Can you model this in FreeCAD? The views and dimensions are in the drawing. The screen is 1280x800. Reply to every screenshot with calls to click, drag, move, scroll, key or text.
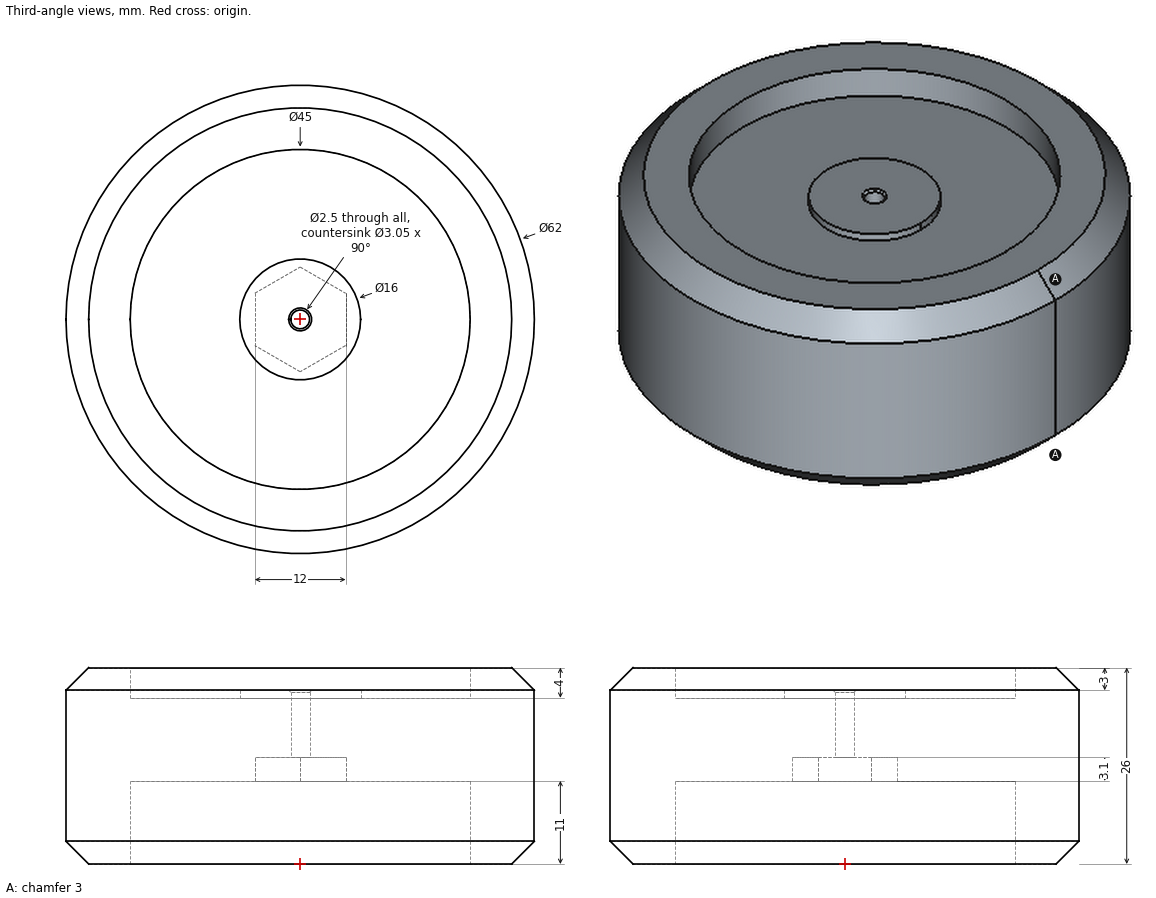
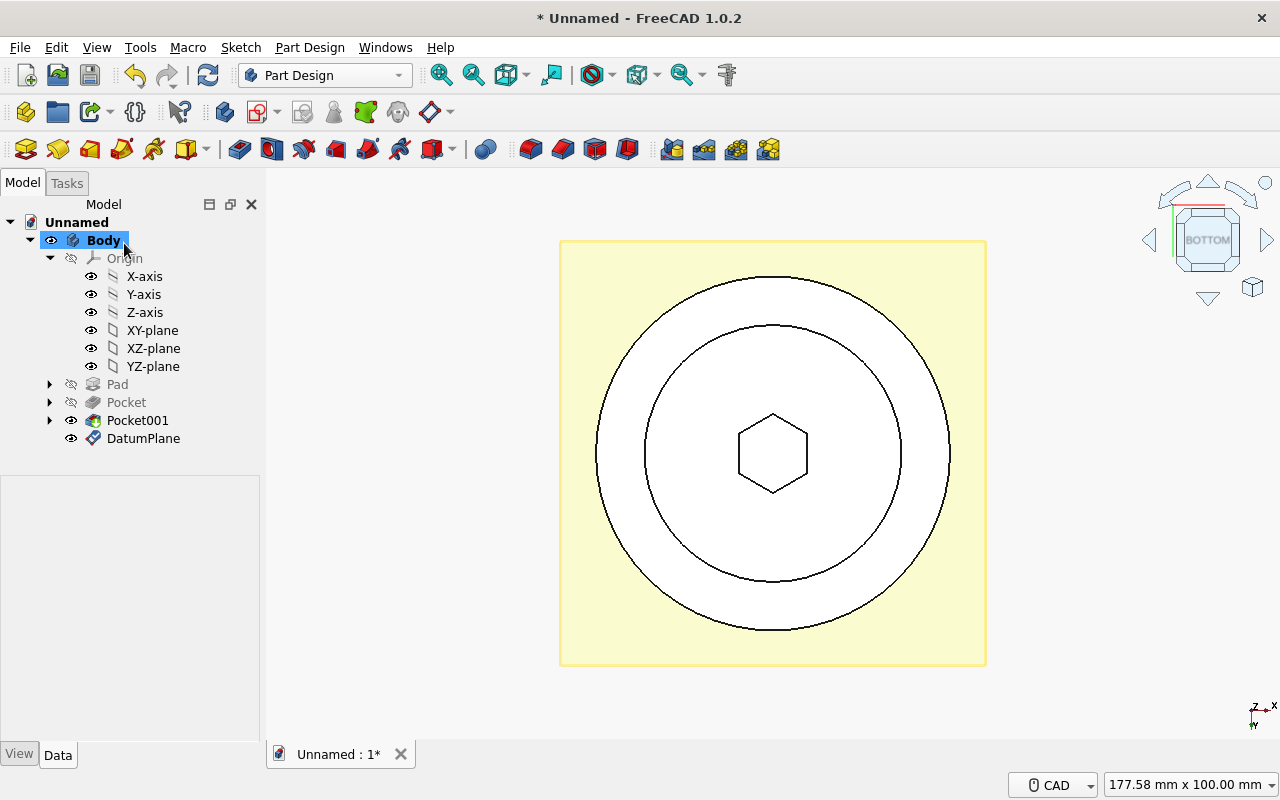
click(116, 438)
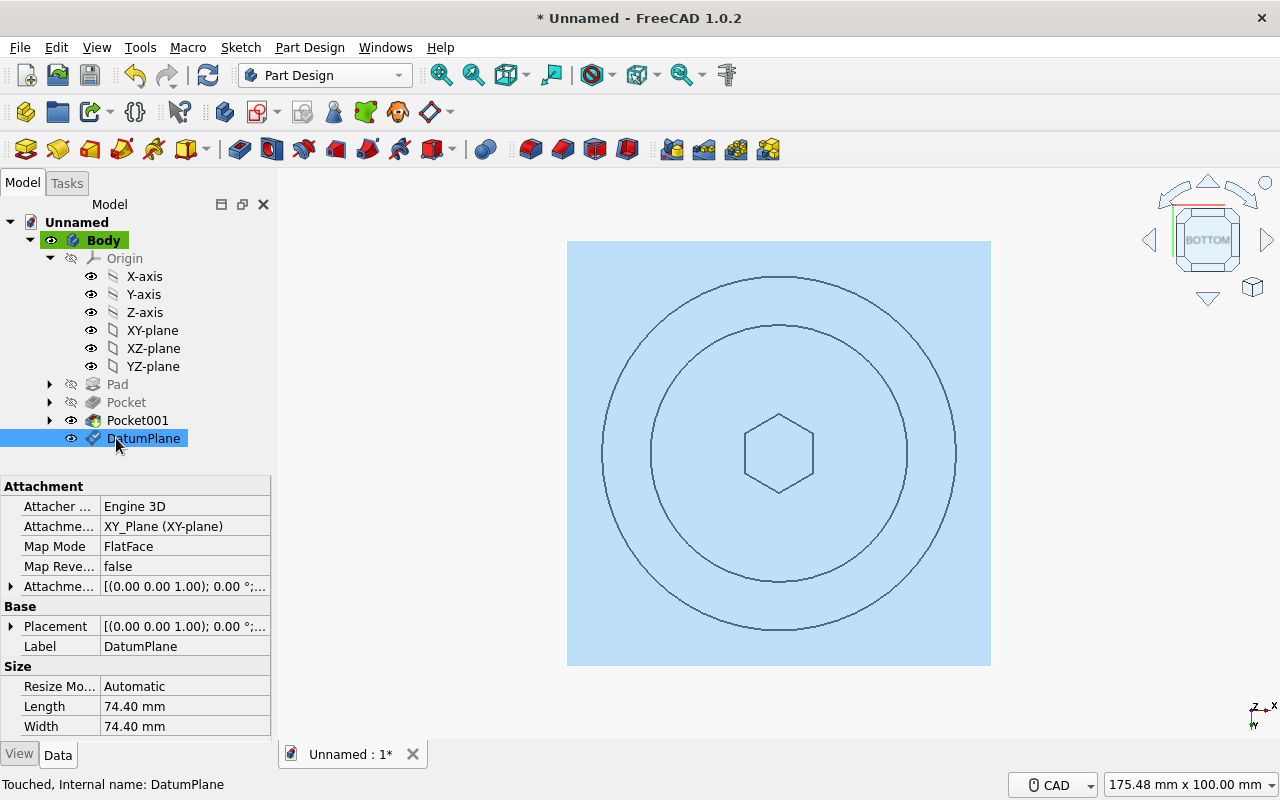
click(258, 112)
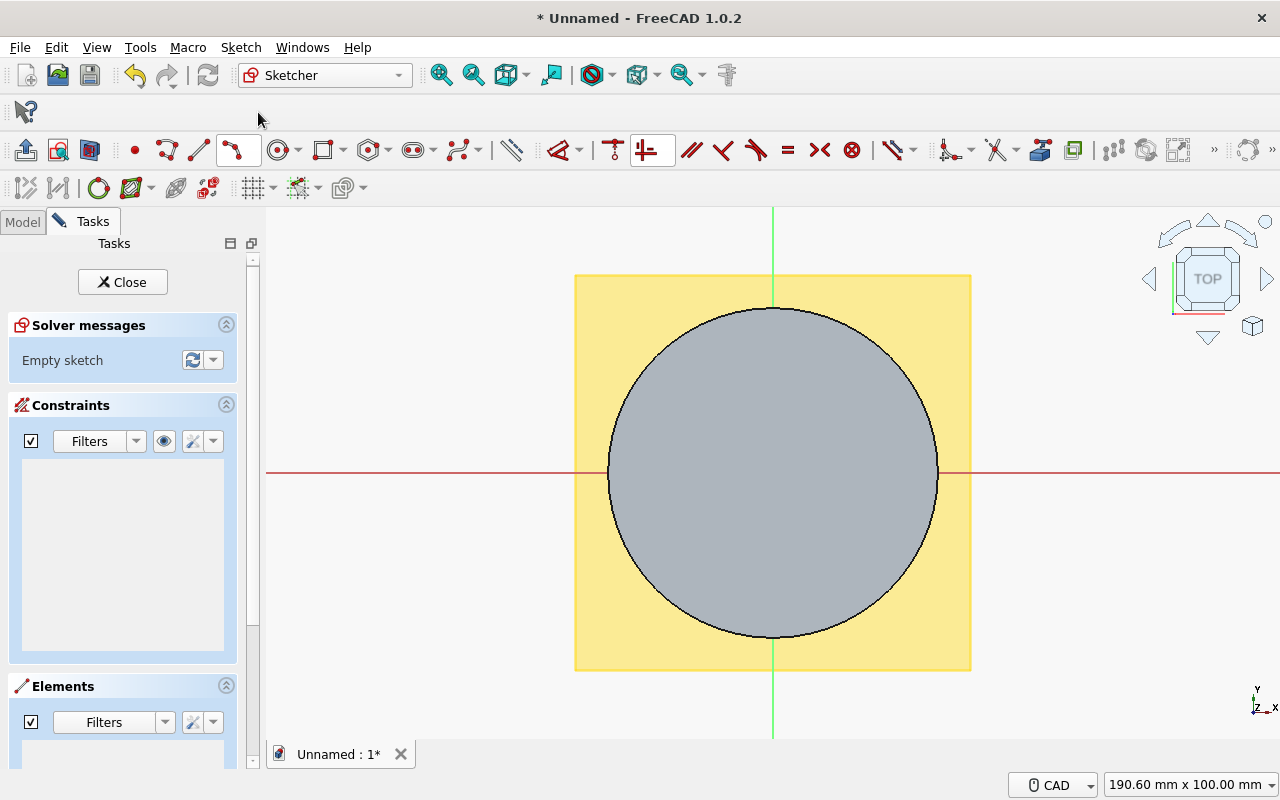
click(90, 150)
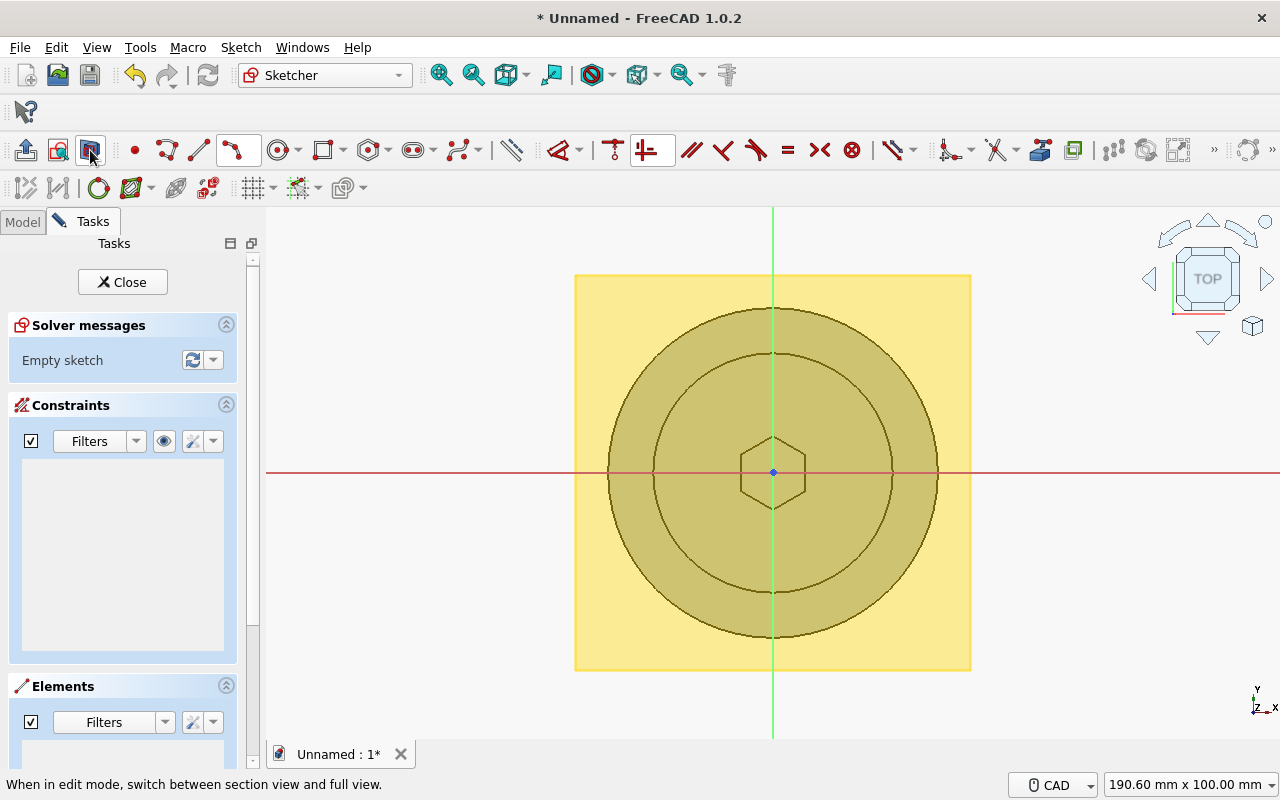
scroll(912, 473, up, 2)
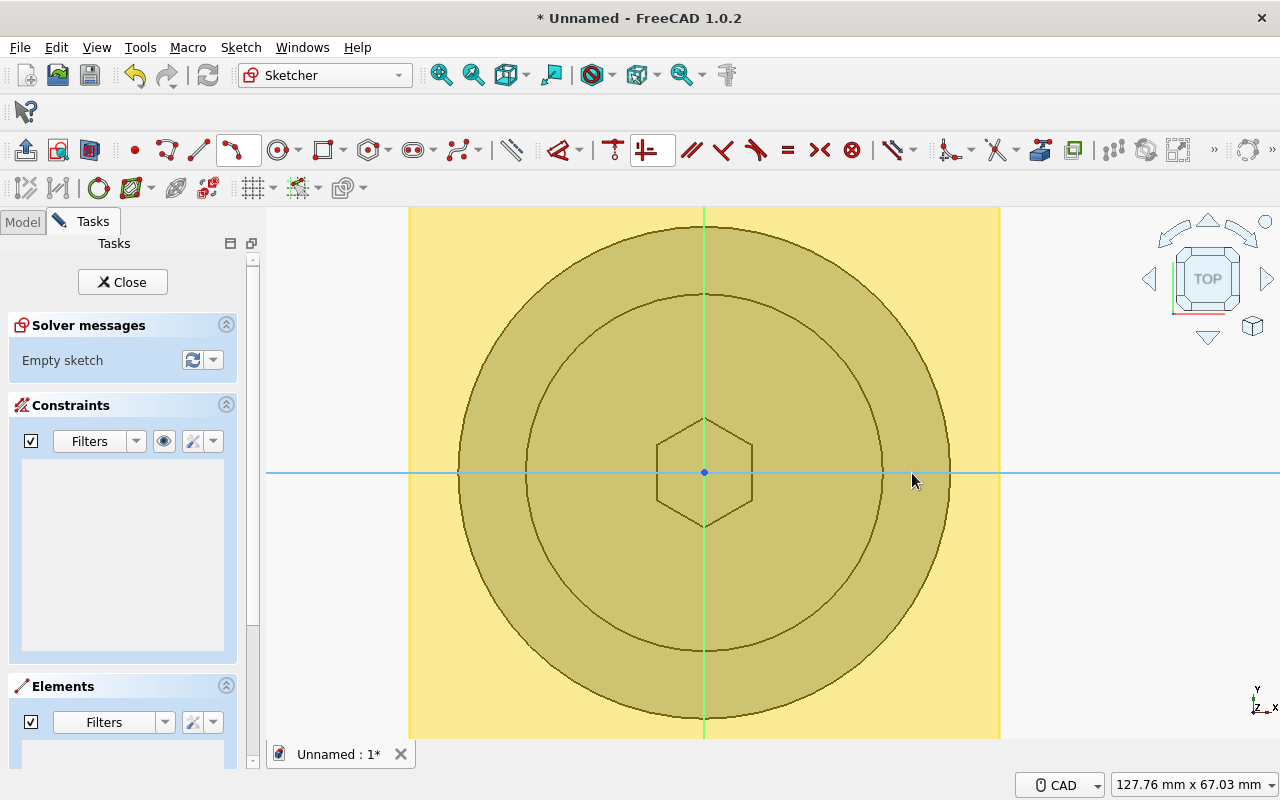
click(278, 150)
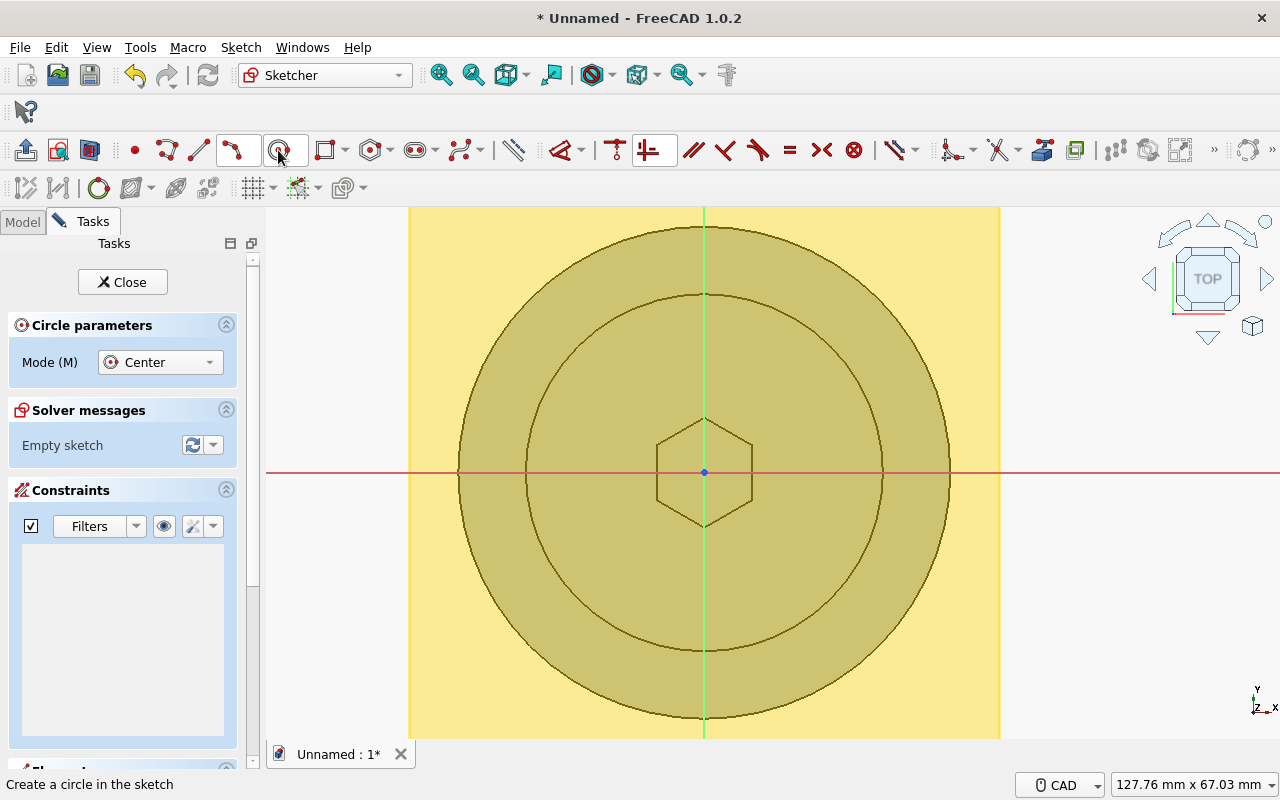
click(704, 473)
click(831, 346)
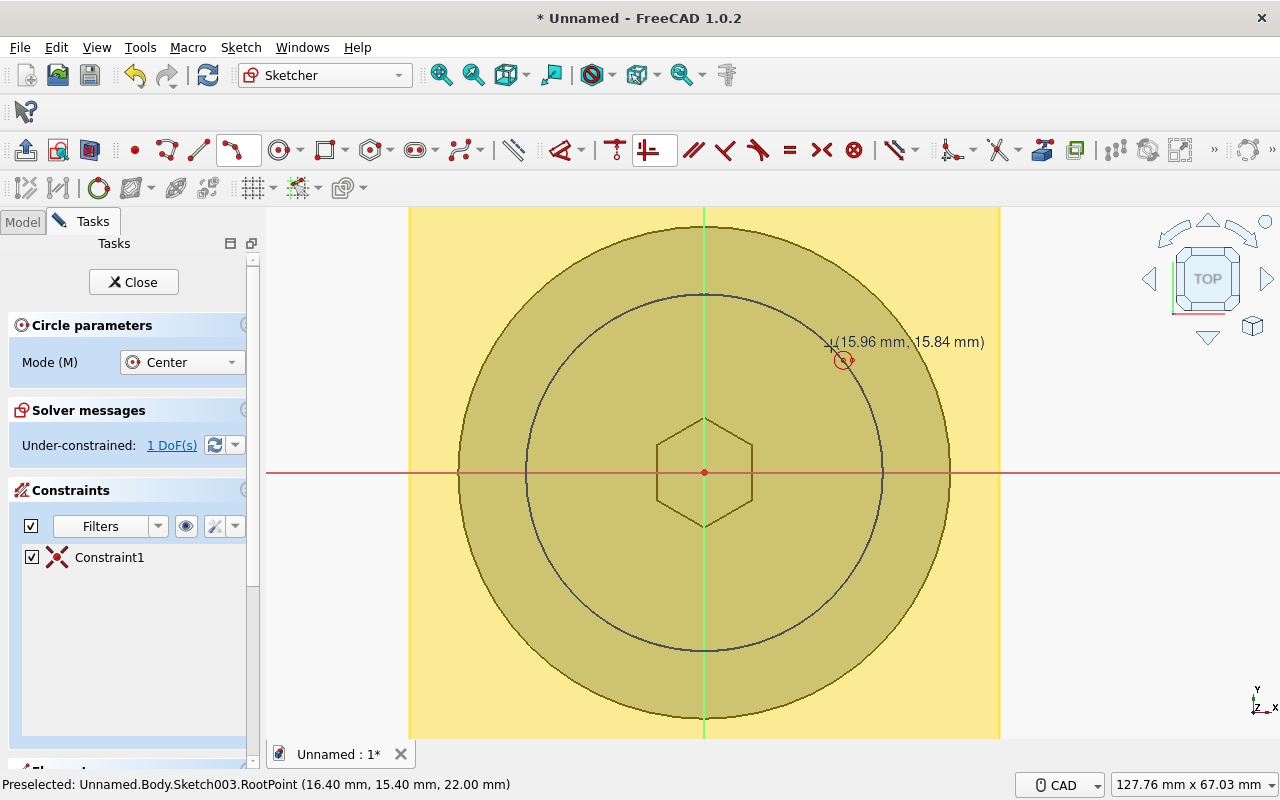
click(704, 473)
click(749, 428)
key(Escape)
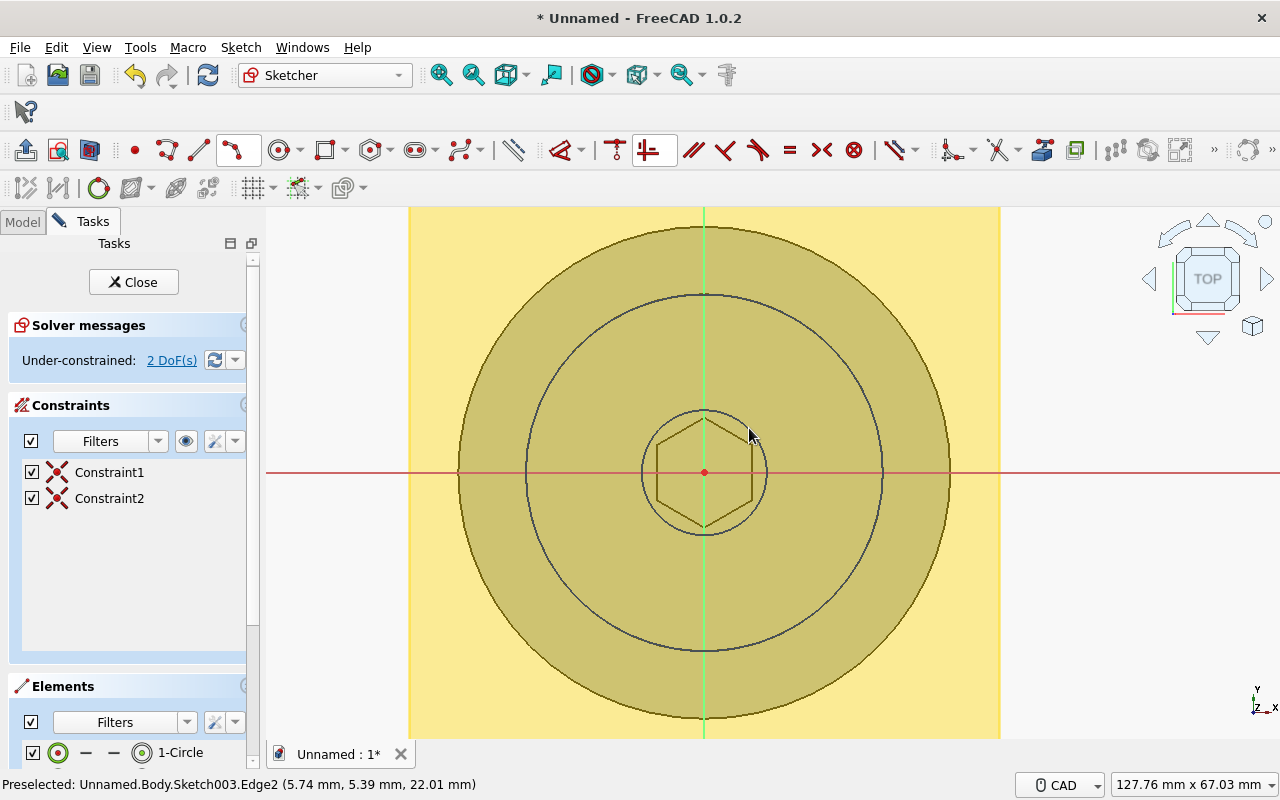
click(560, 150)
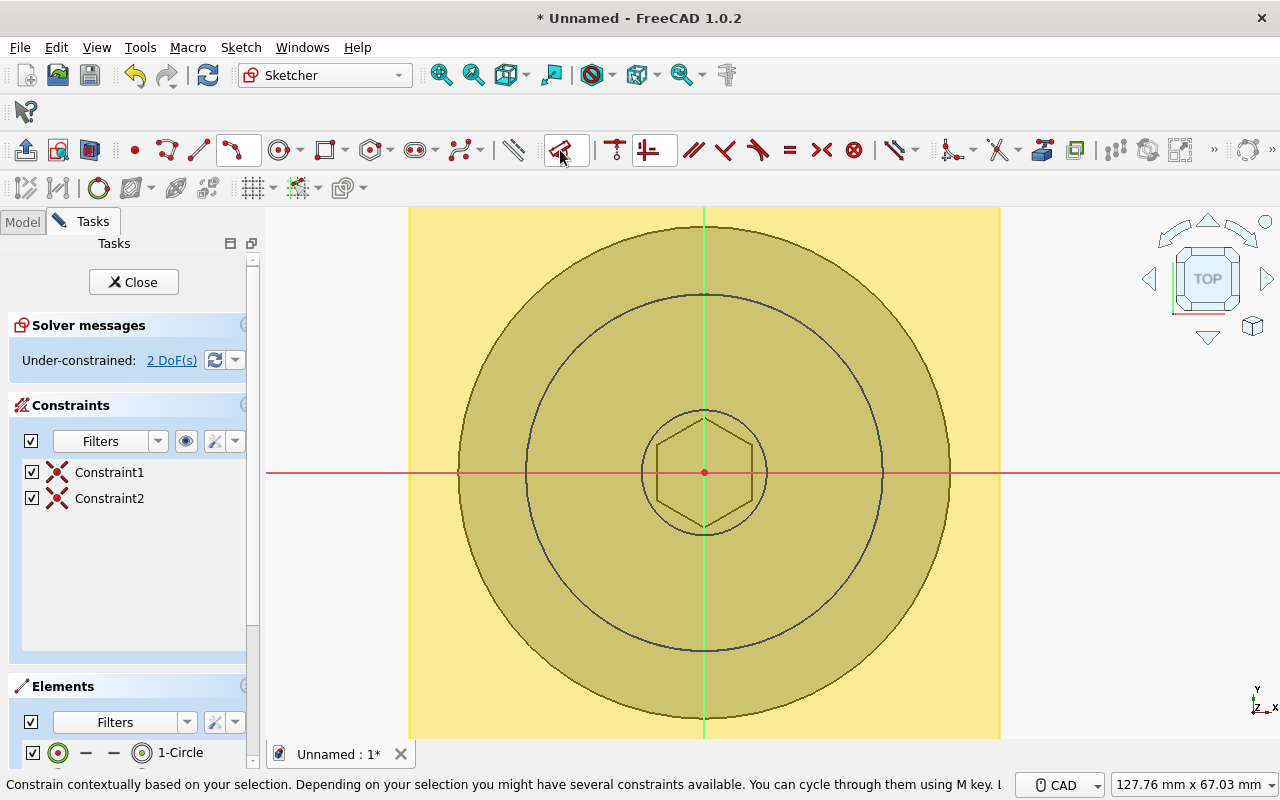
click(830, 346)
click(853, 323)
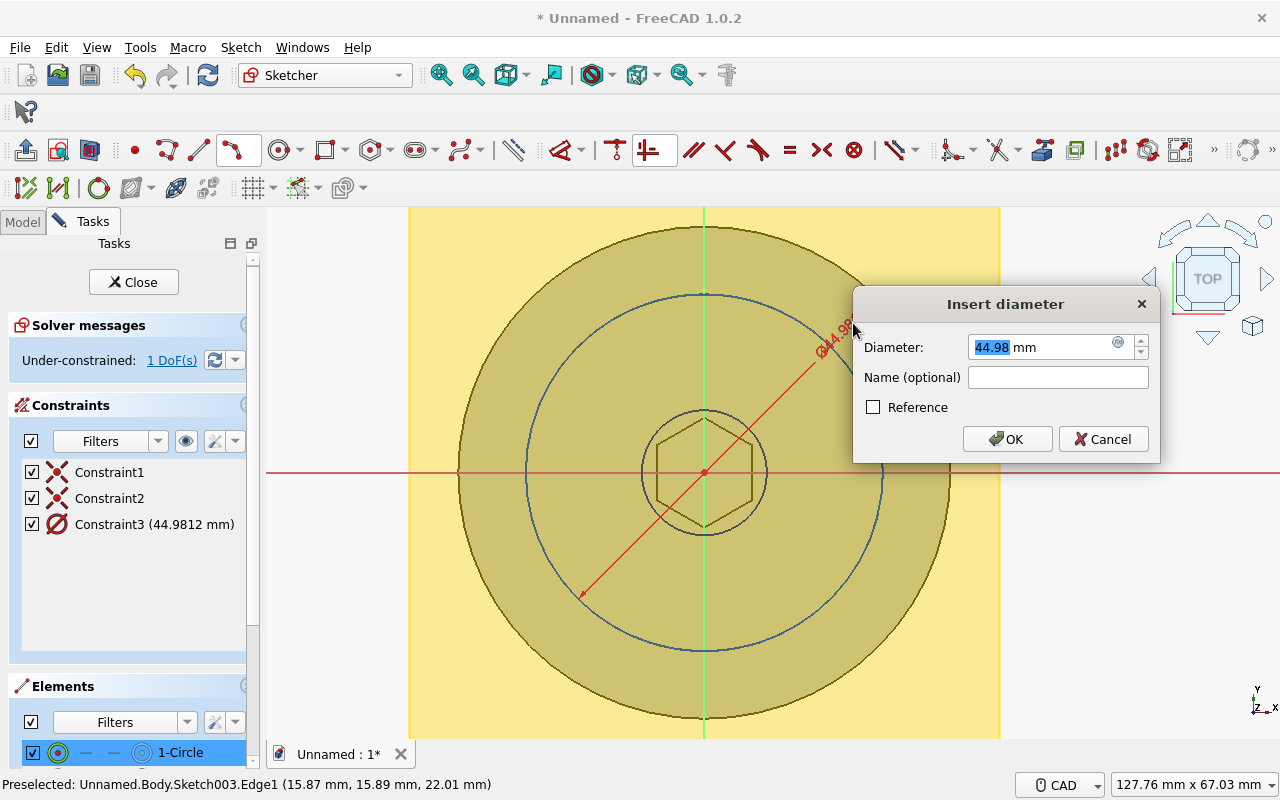
text(45)
key(Return)